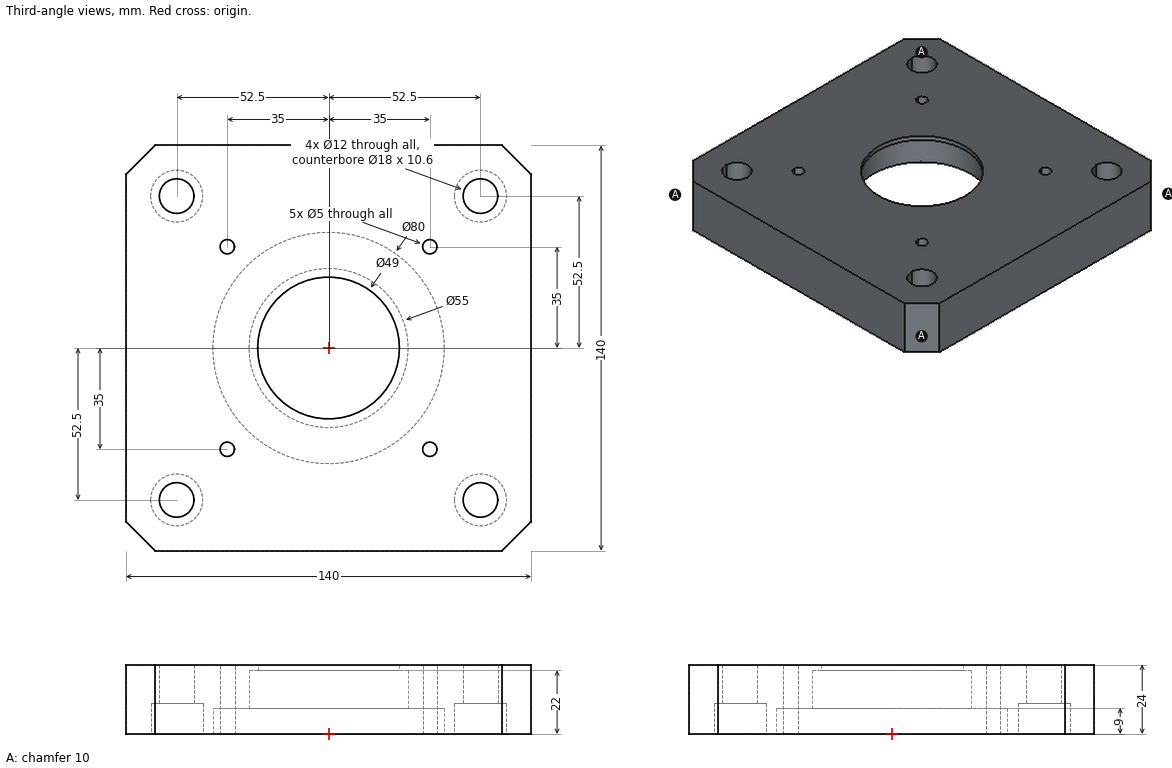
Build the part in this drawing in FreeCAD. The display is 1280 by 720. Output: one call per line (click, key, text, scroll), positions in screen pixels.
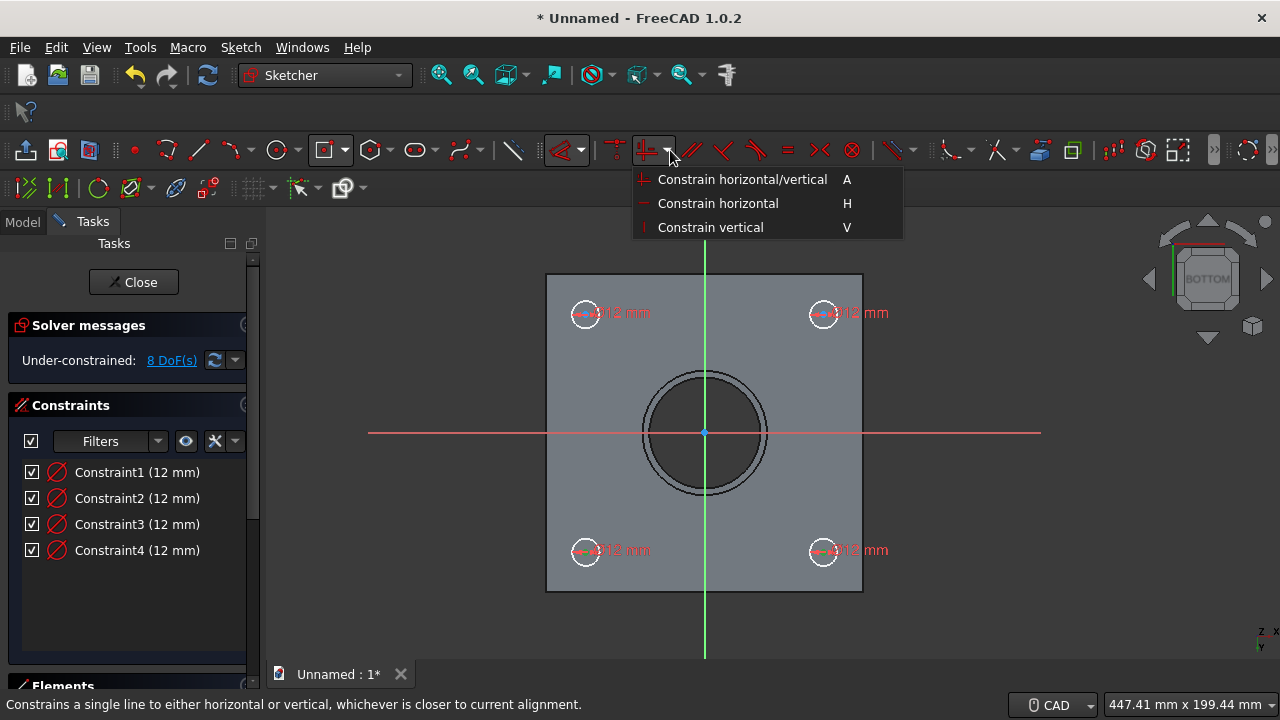
click(768, 203)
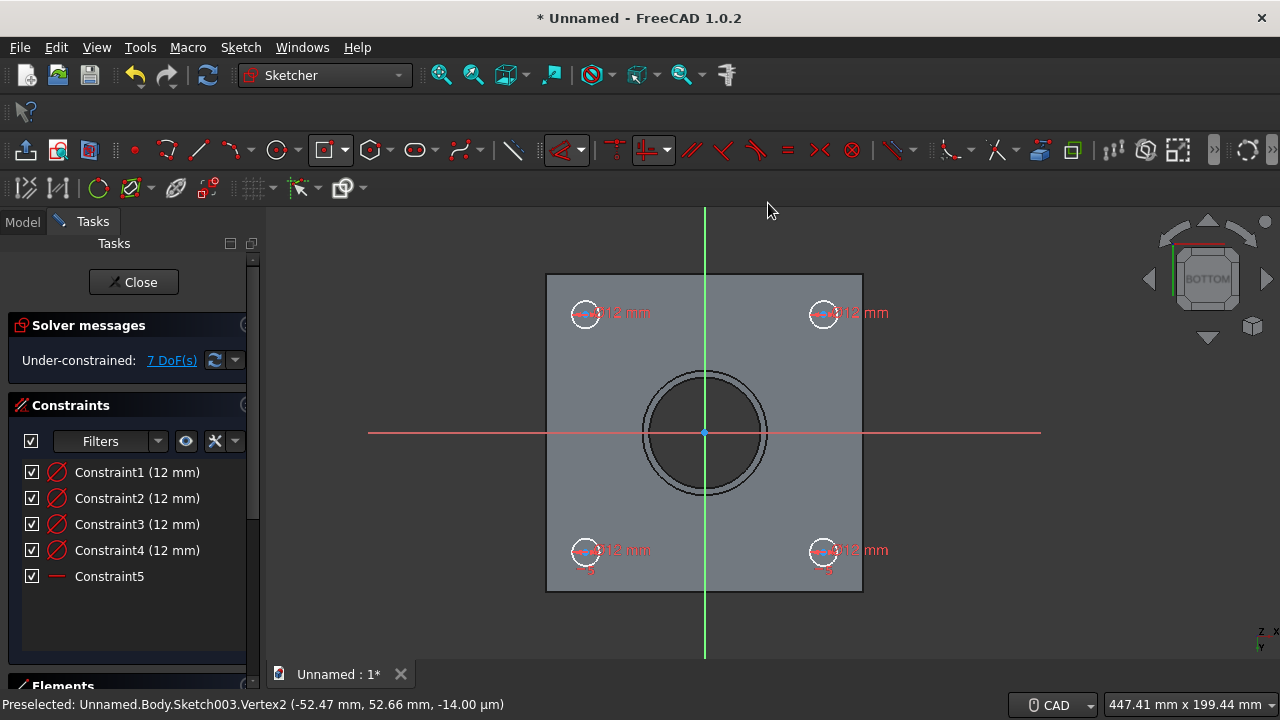
click(586, 552)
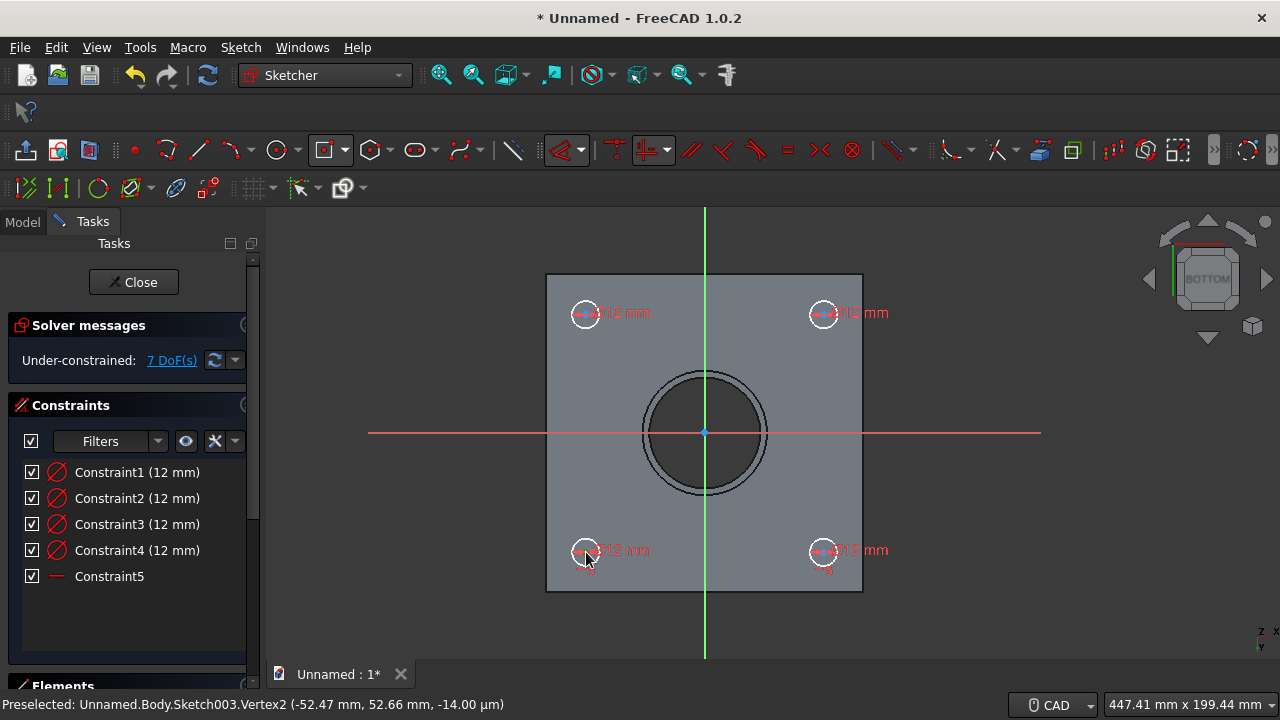
click(586, 315)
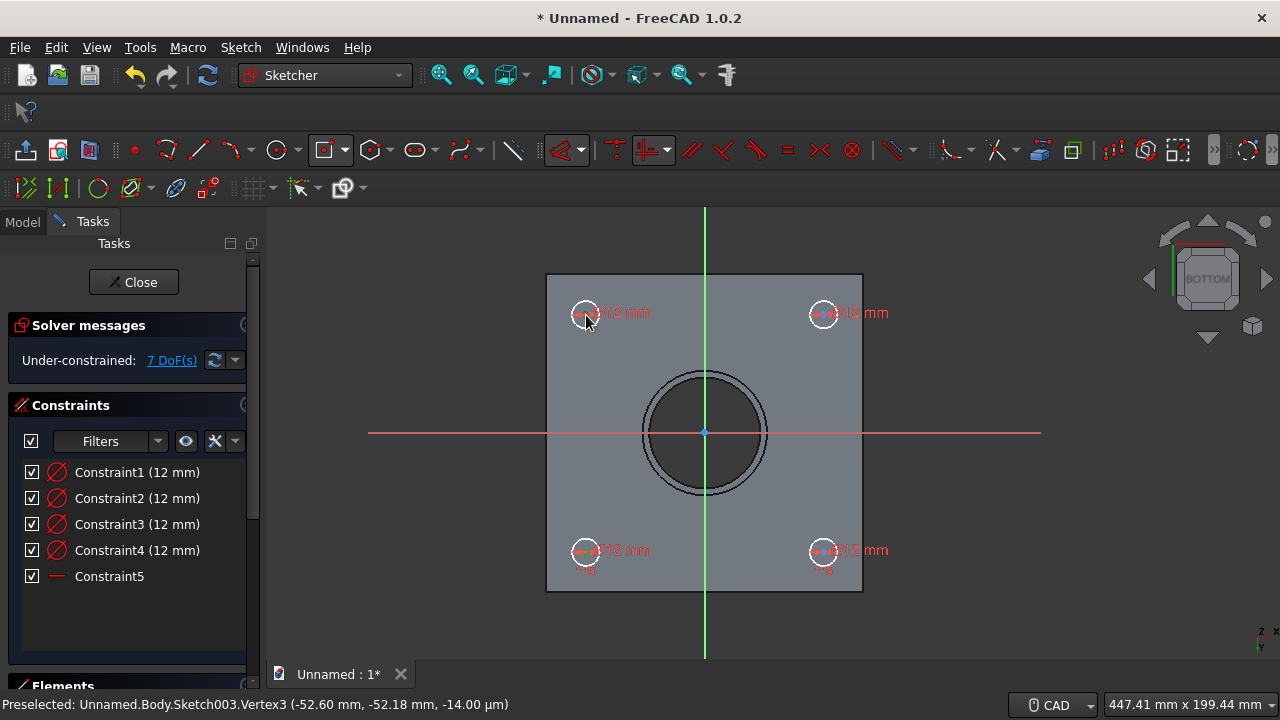
click(670, 150)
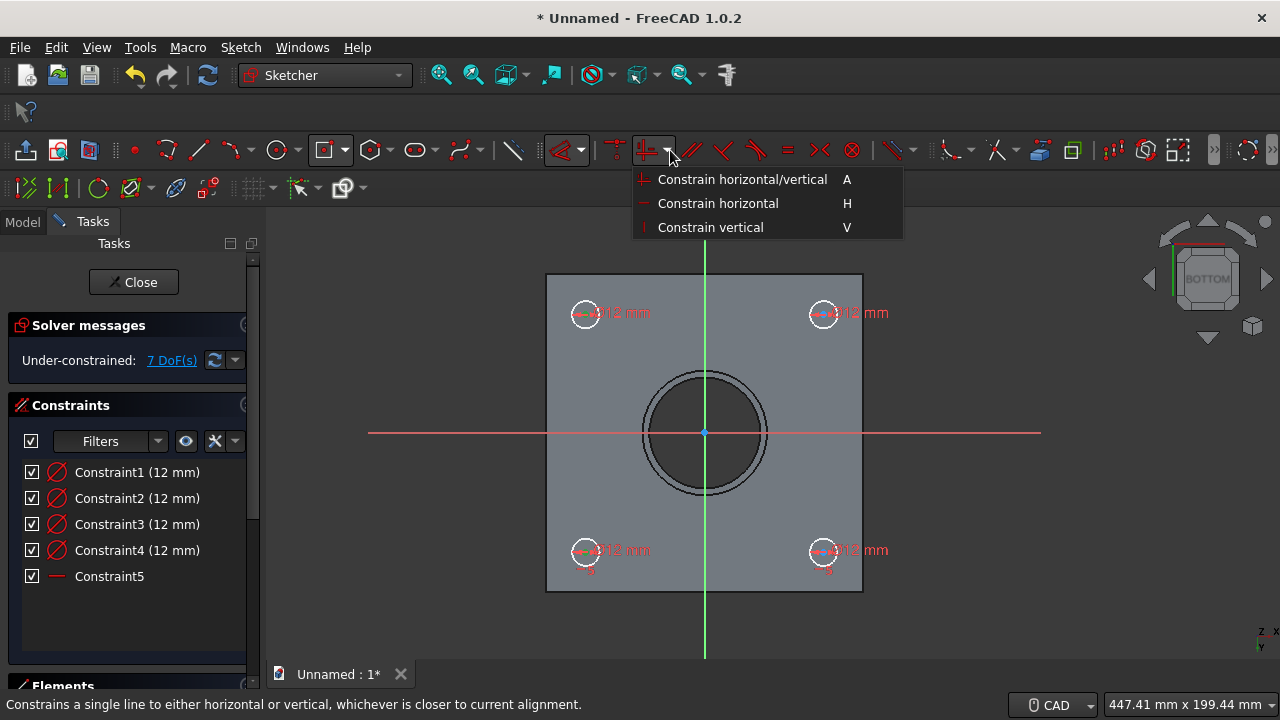
click(768, 227)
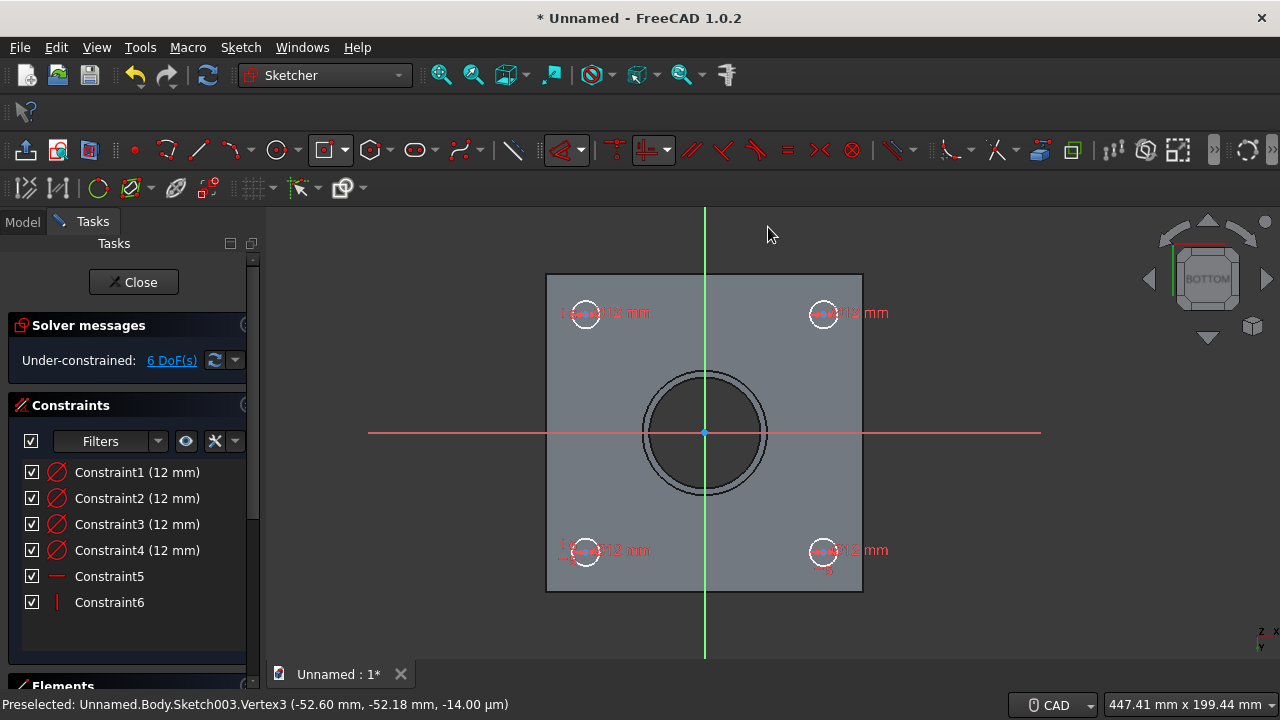
click(824, 552)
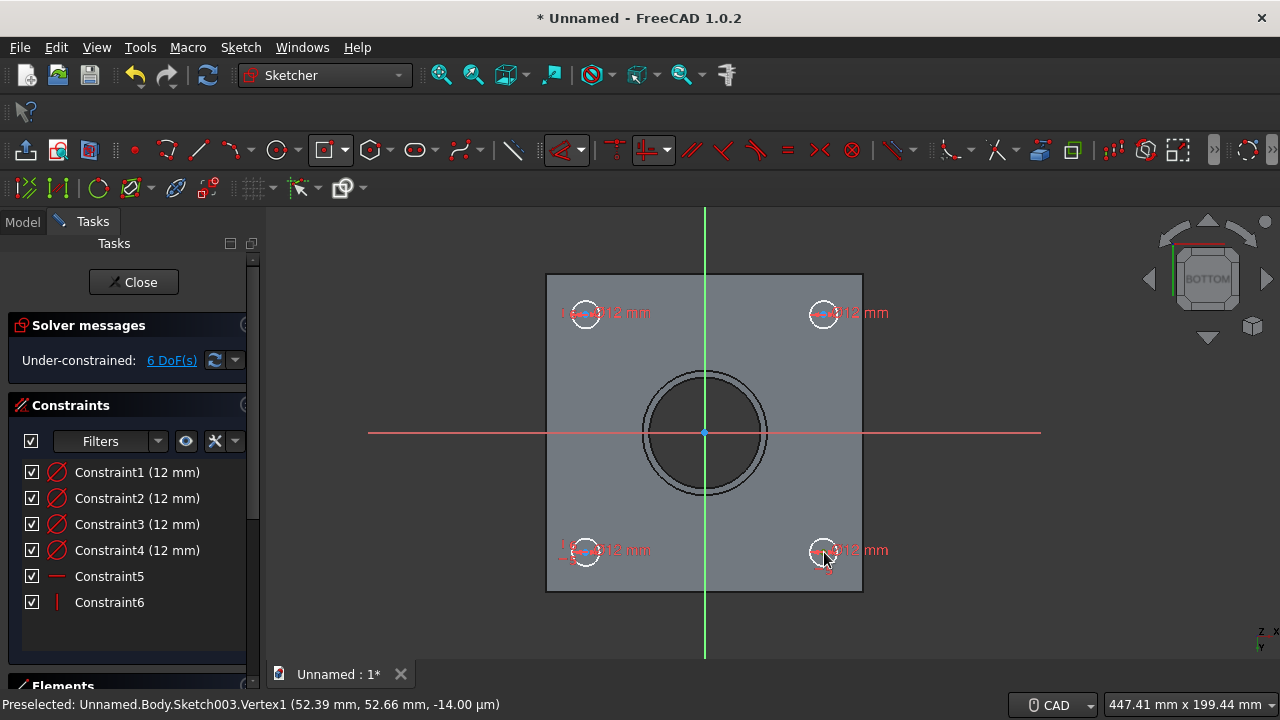
click(824, 315)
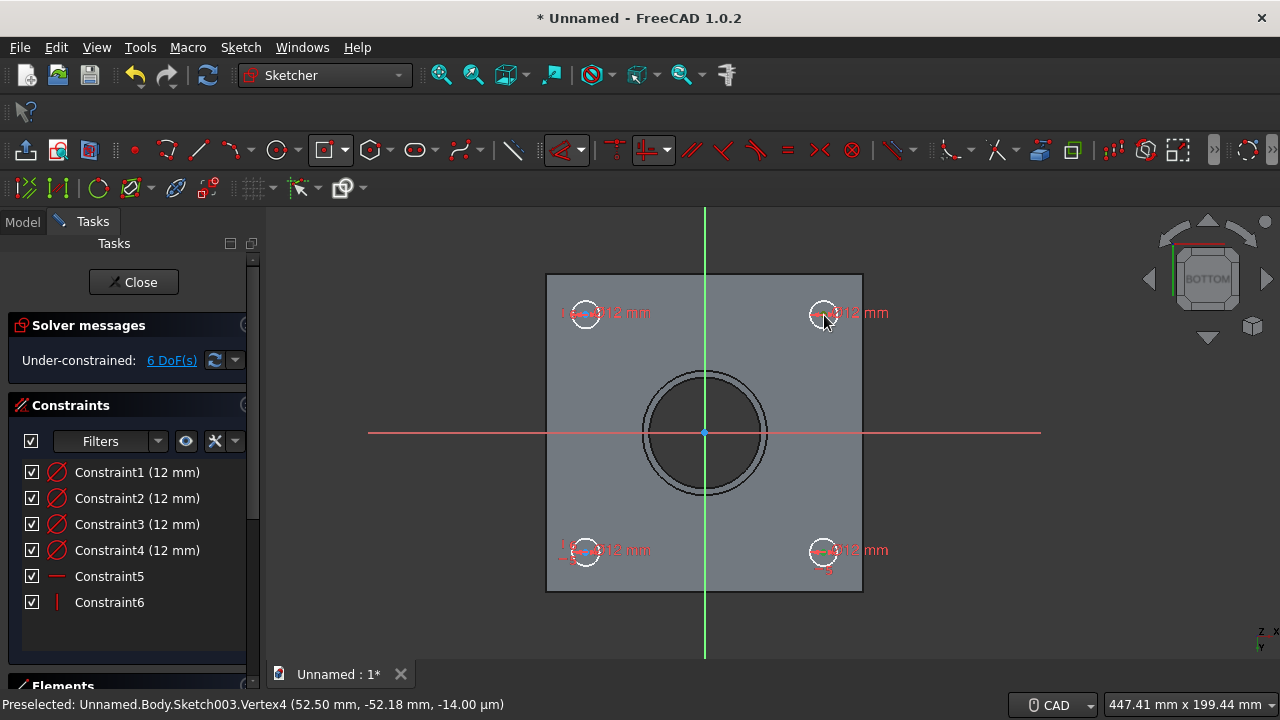
click(670, 150)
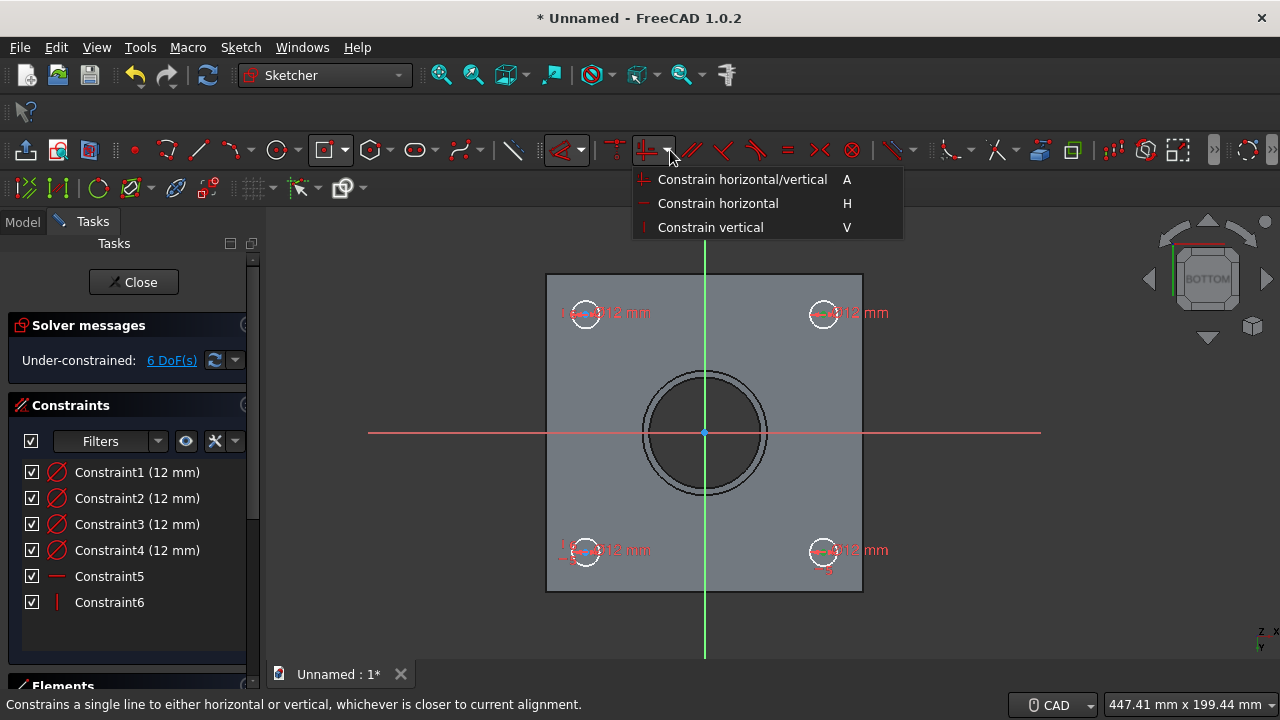
click(768, 227)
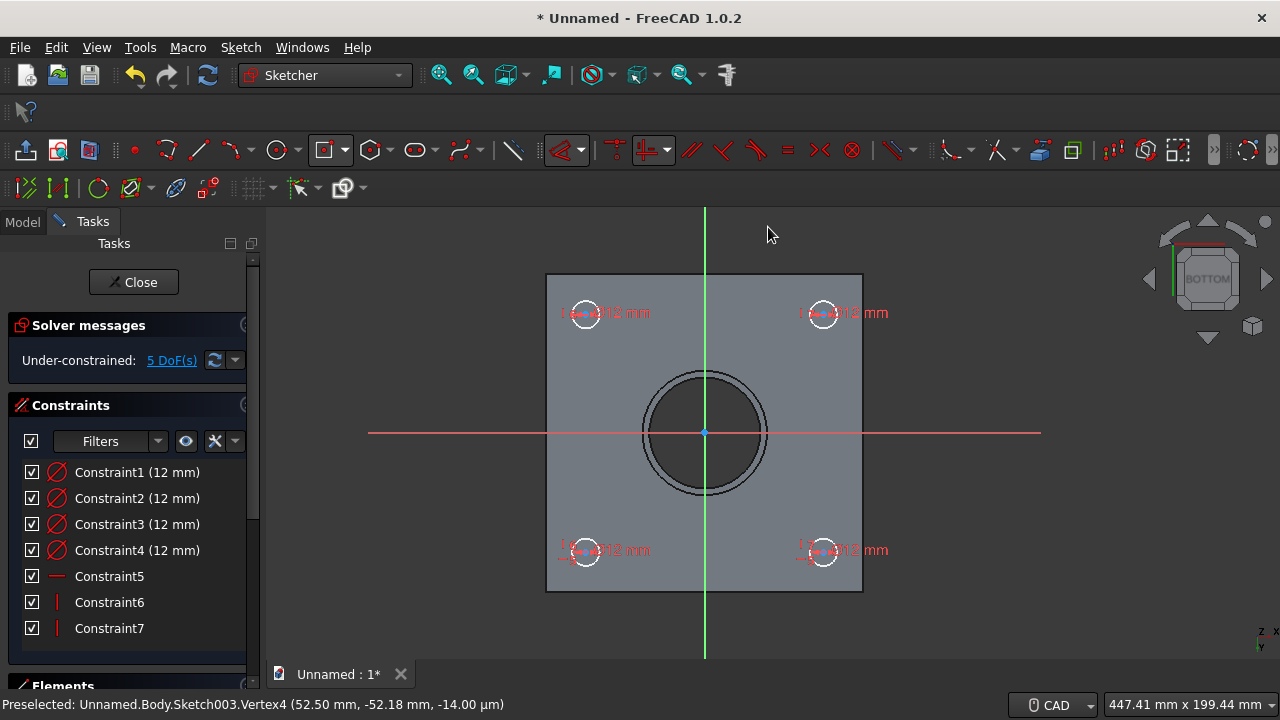
click(586, 315)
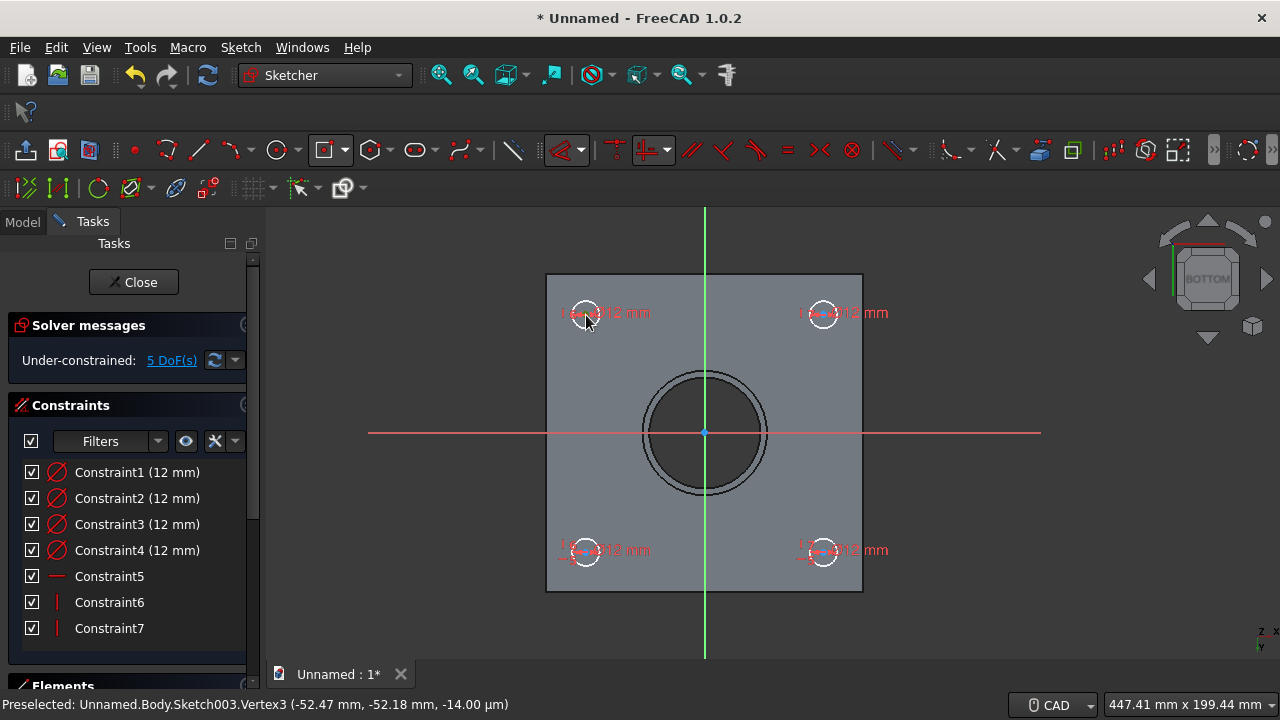
click(824, 315)